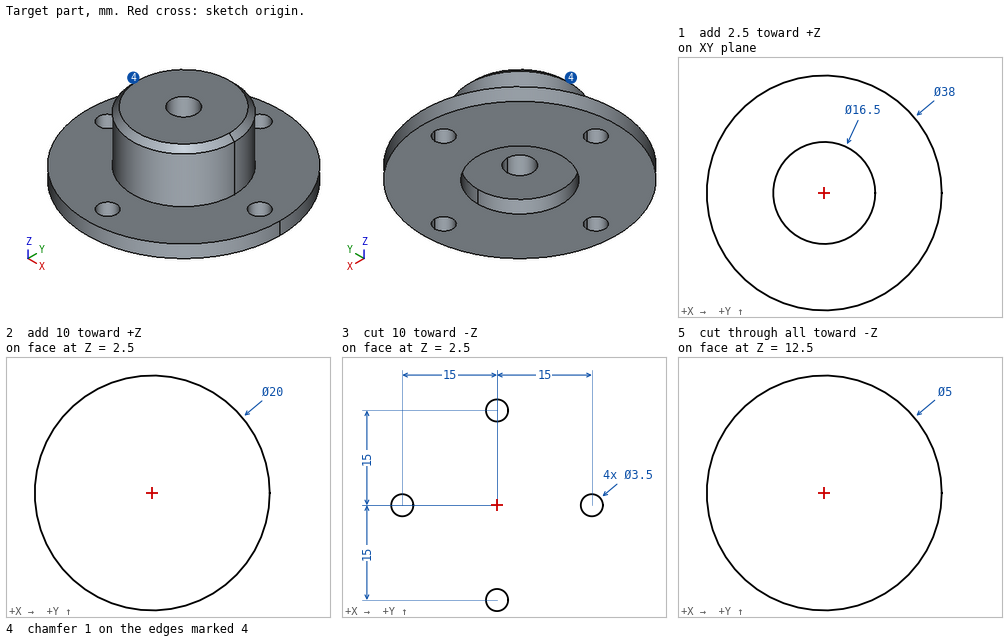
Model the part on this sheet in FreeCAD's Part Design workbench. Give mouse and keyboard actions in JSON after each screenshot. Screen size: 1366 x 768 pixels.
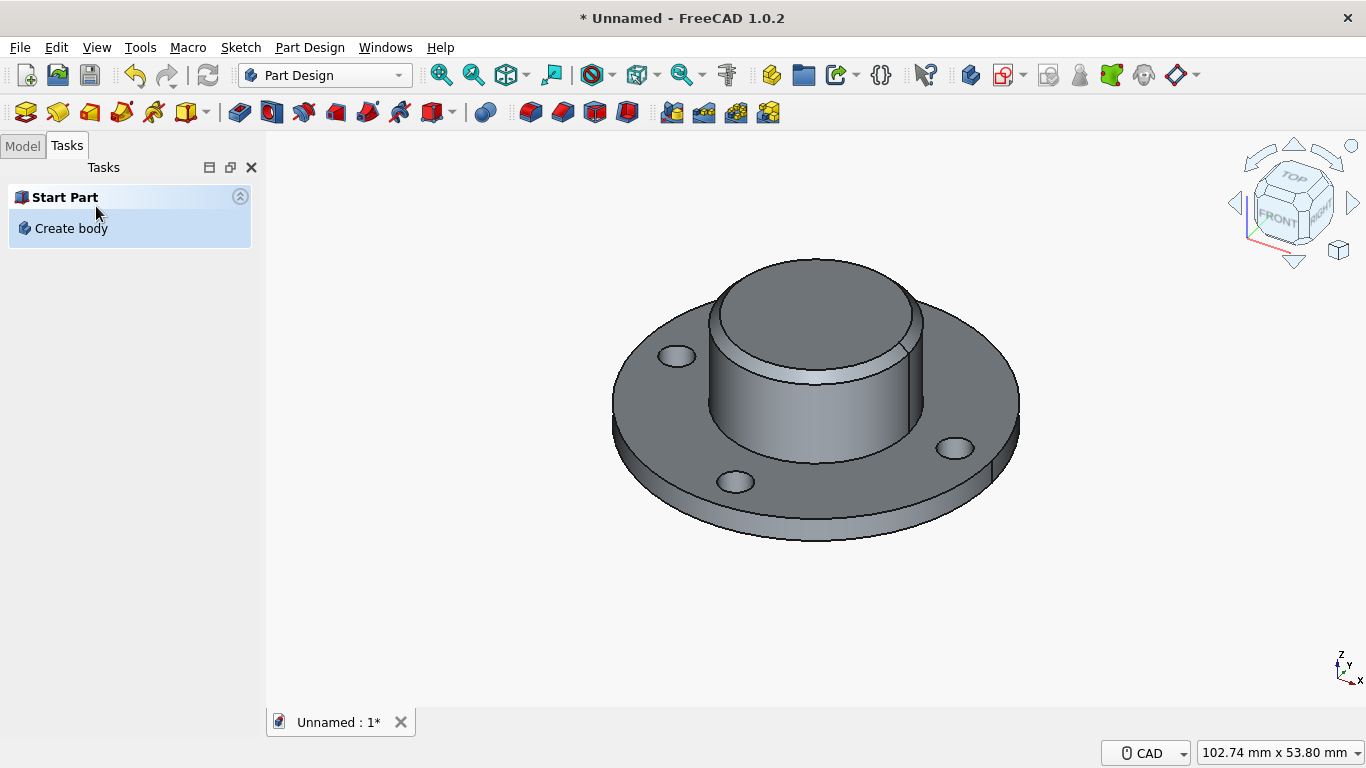
{"action": "left_click", "coordinate": [816, 314]}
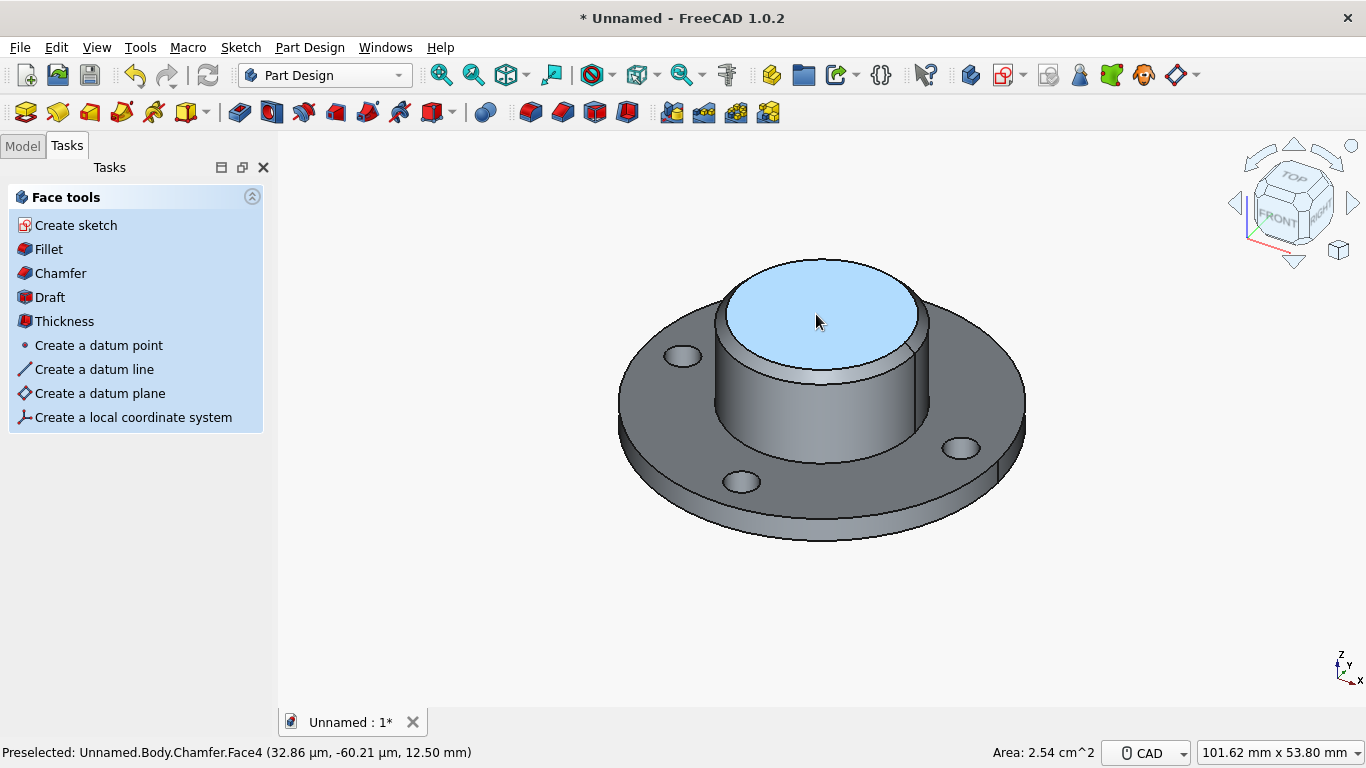
{"action": "left_click", "coordinate": [1004, 76]}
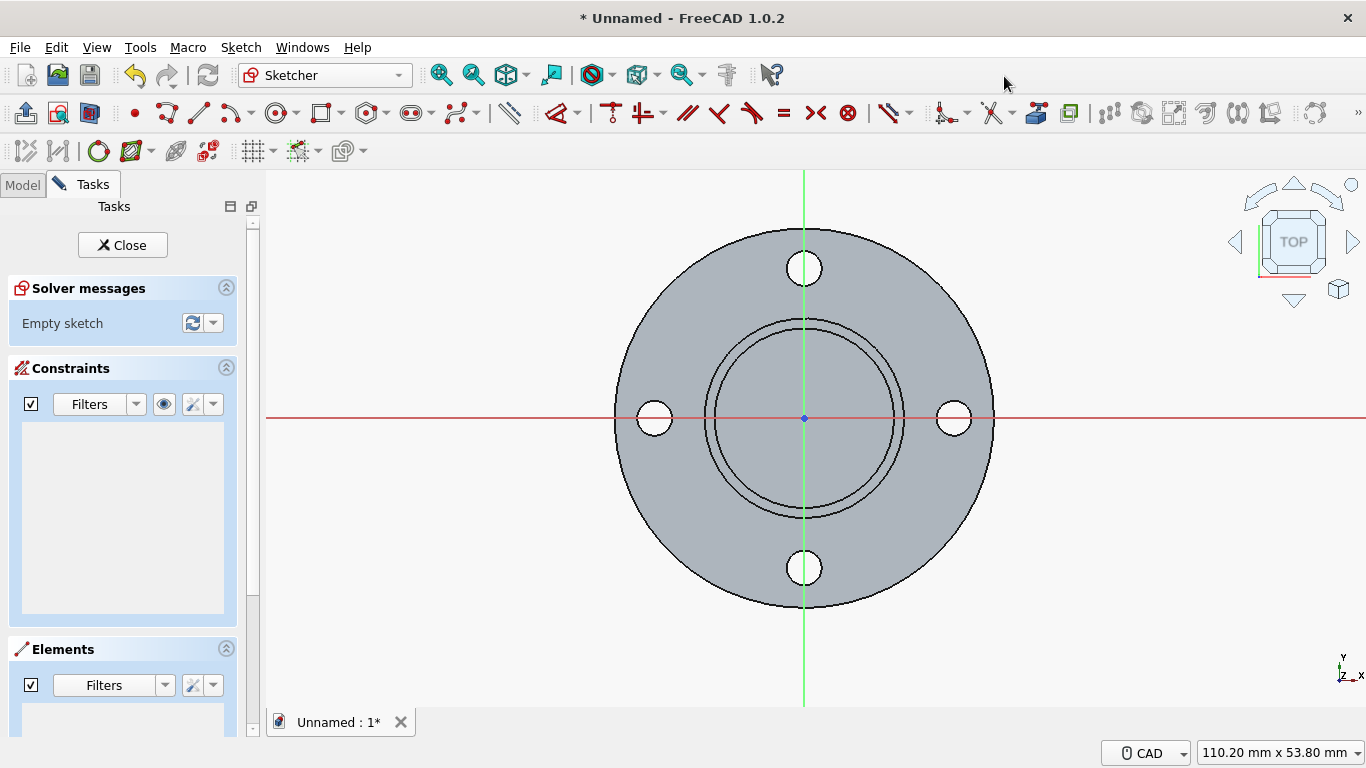
{"action": "scroll", "coordinate": [813, 415], "scroll_direction": "up", "scroll_amount": 10}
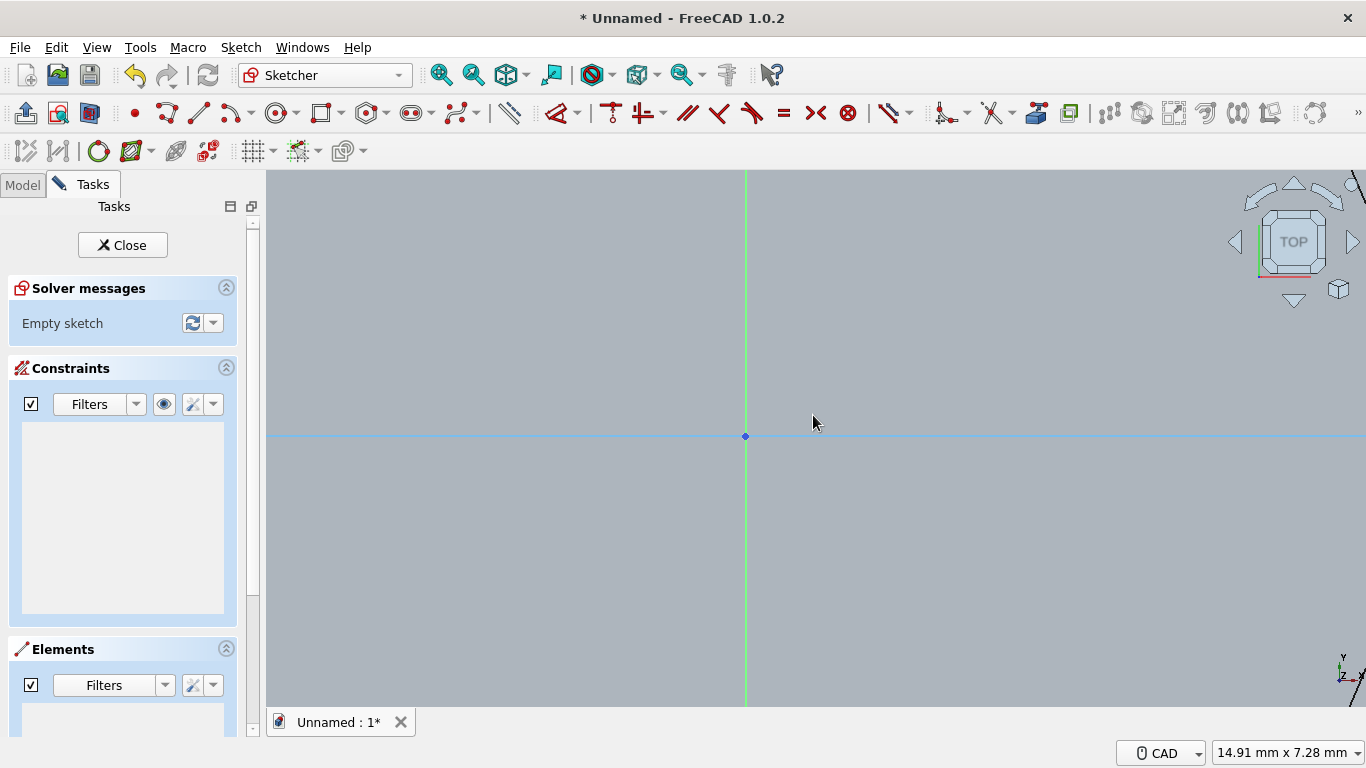
{"action": "key", "text": "g c"}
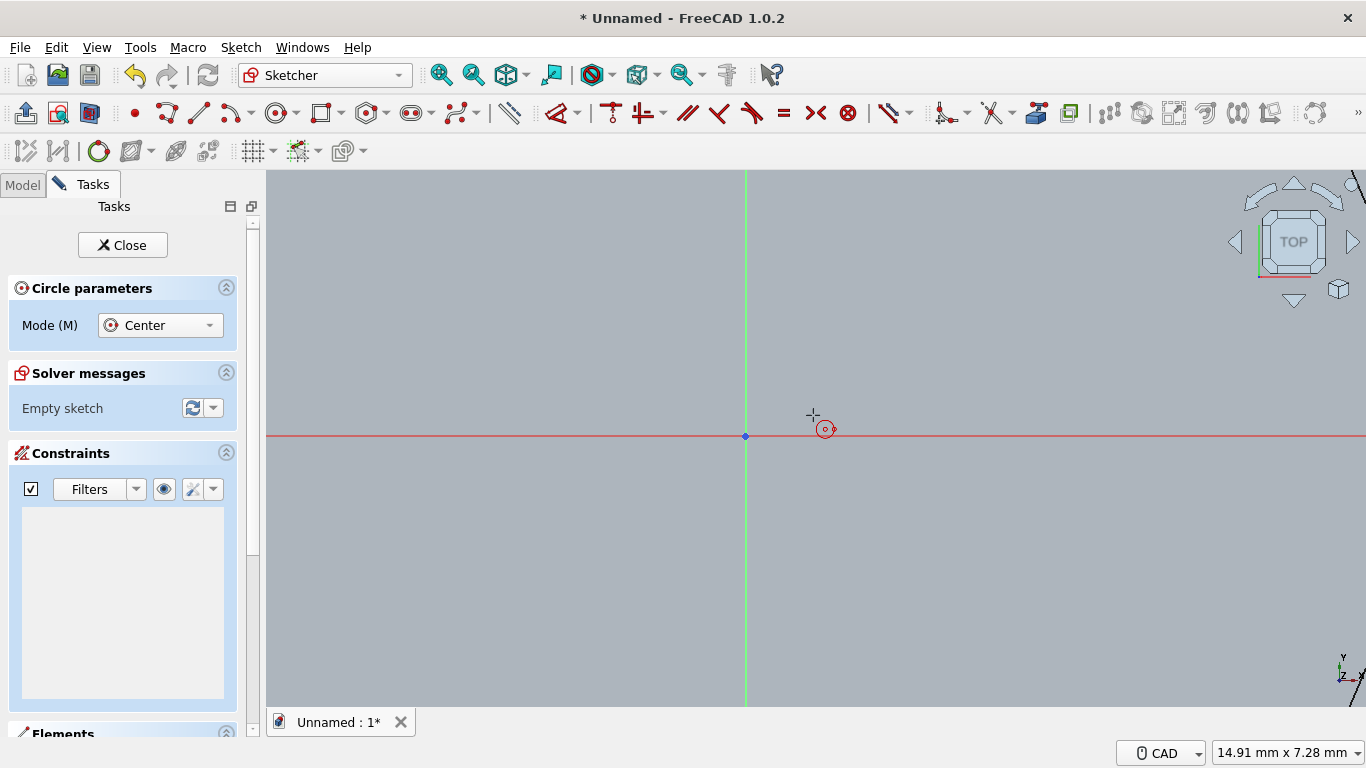
{"action": "left_click", "coordinate": [746, 436]}
{"action": "mouse_move", "coordinate": [876, 306]}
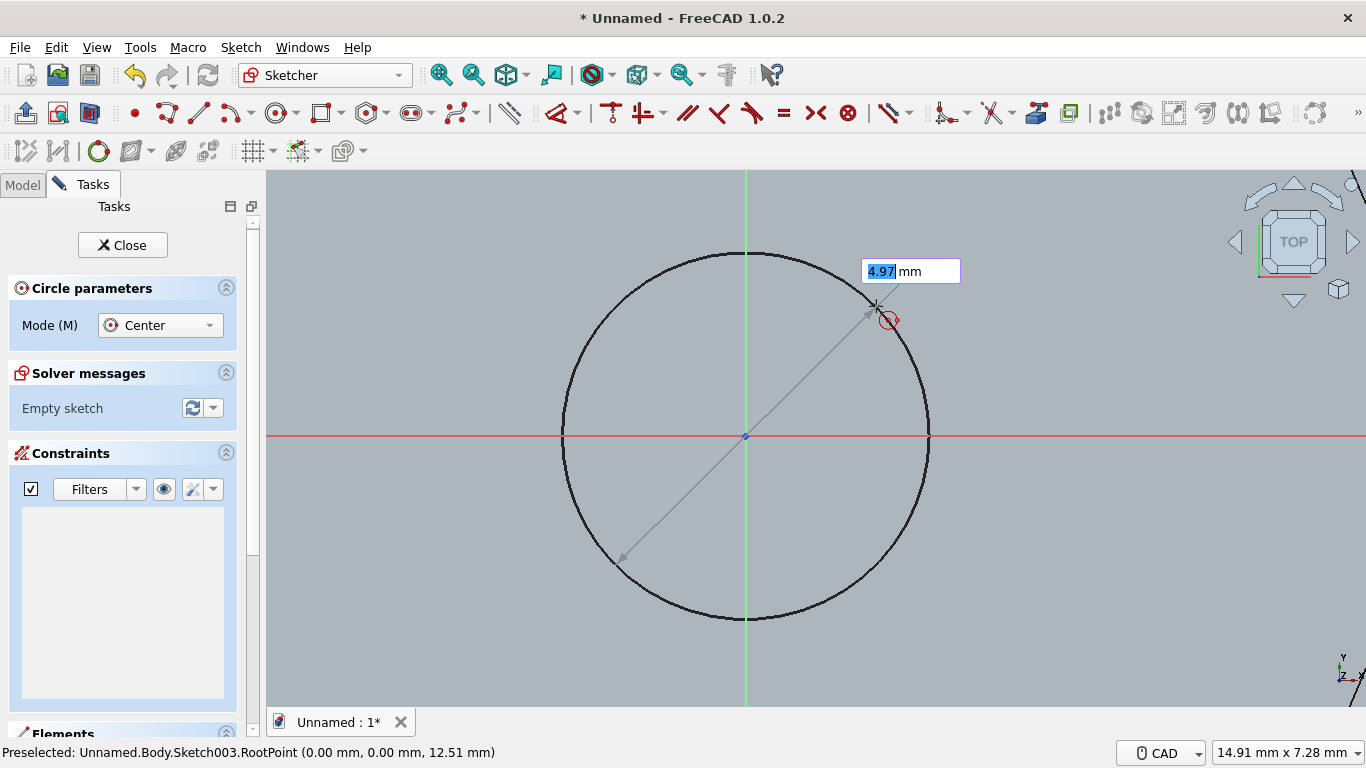
{"action": "type", "text": "5"}
{"action": "key", "text": "Return"}
{"action": "key", "text": "Escape"}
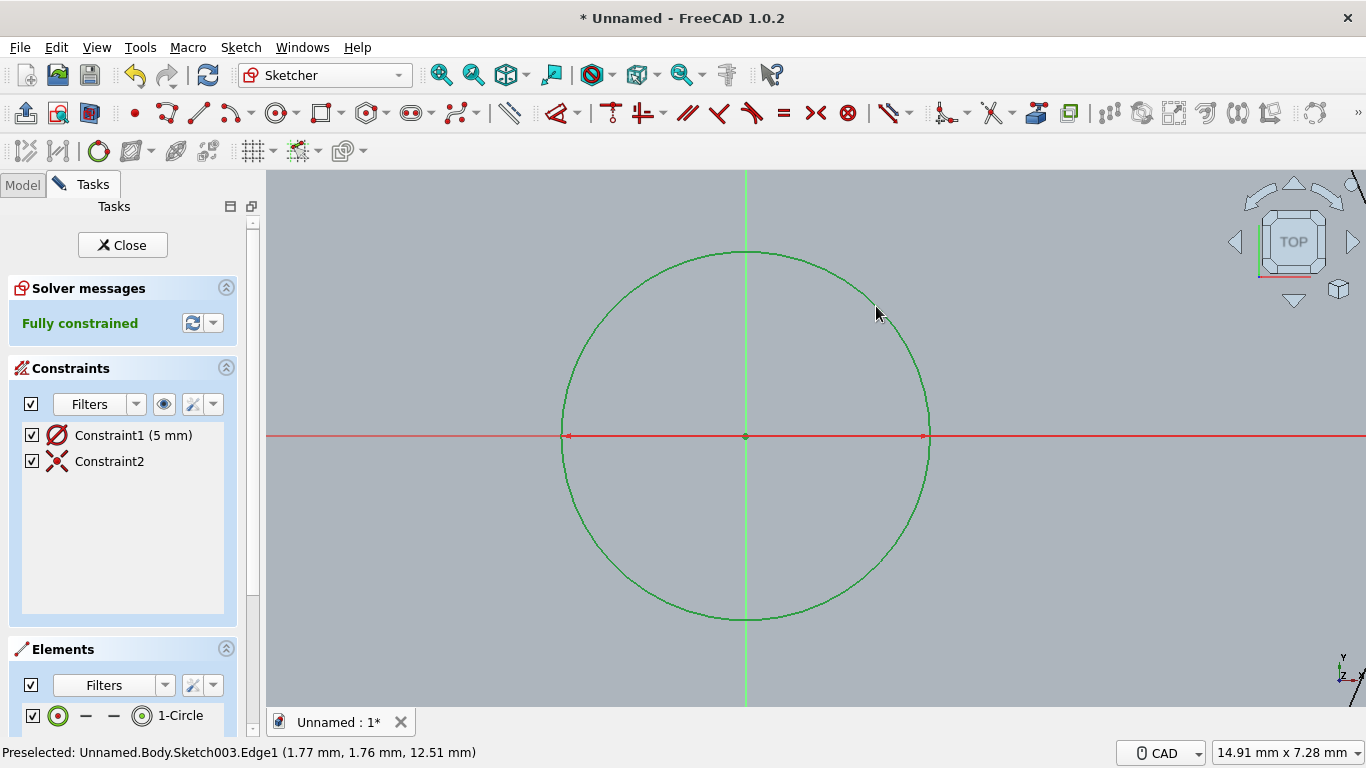
{"action": "left_click", "coordinate": [123, 245]}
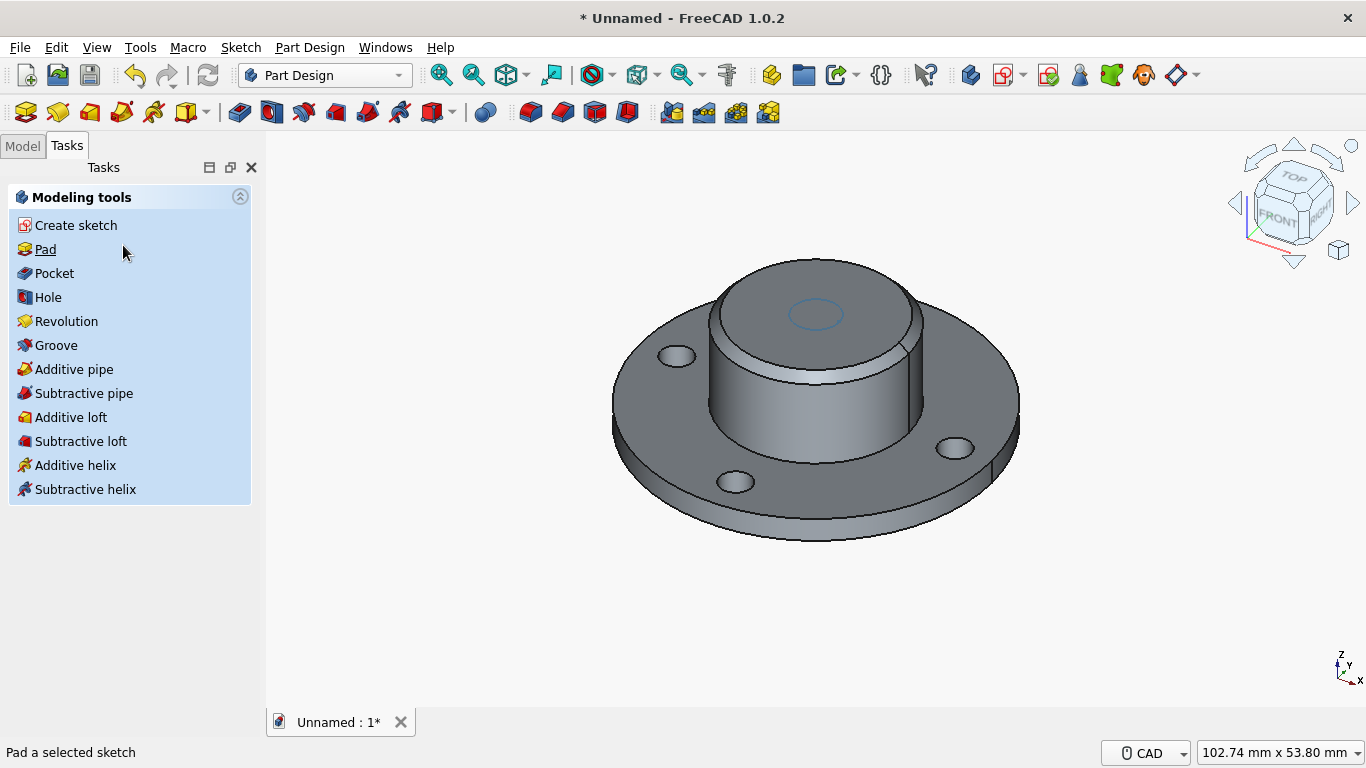
{"action": "left_click", "coordinate": [240, 112]}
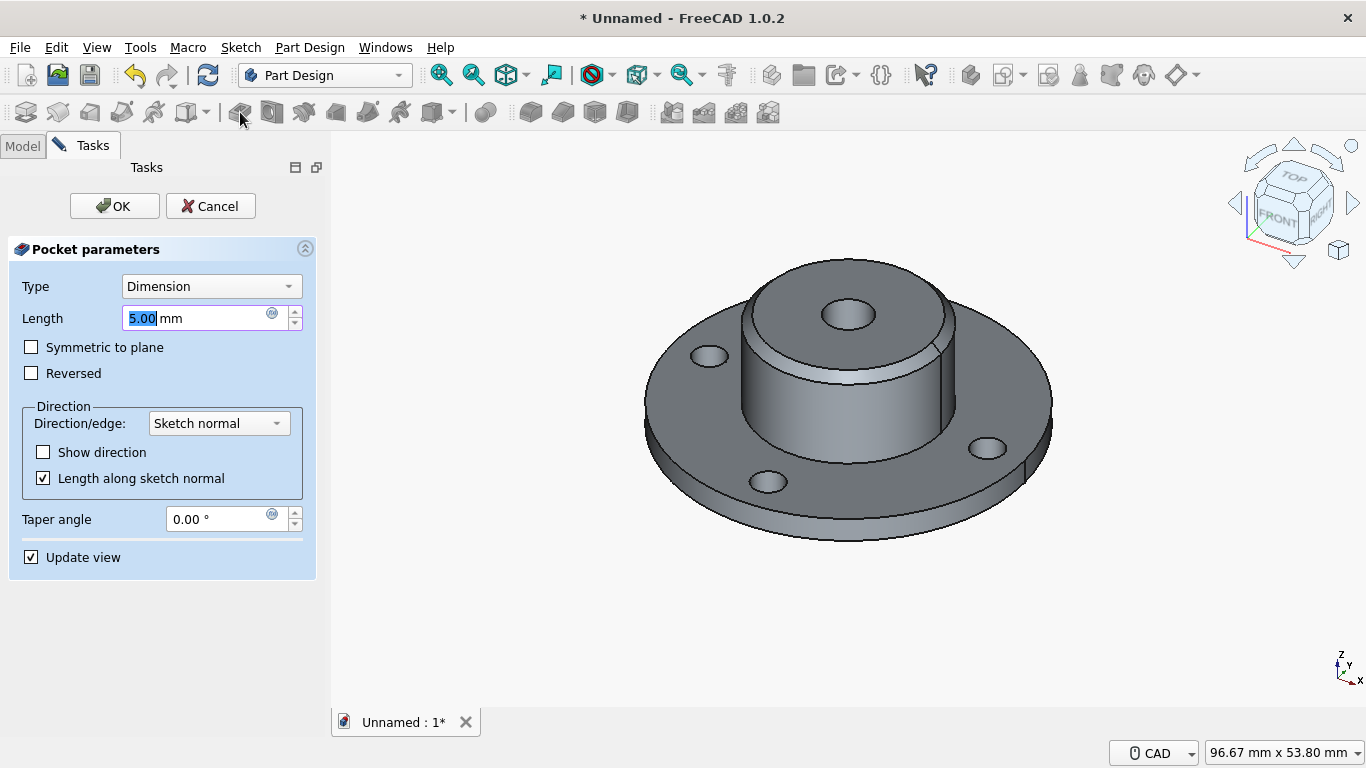
{"action": "left_click", "coordinate": [212, 286]}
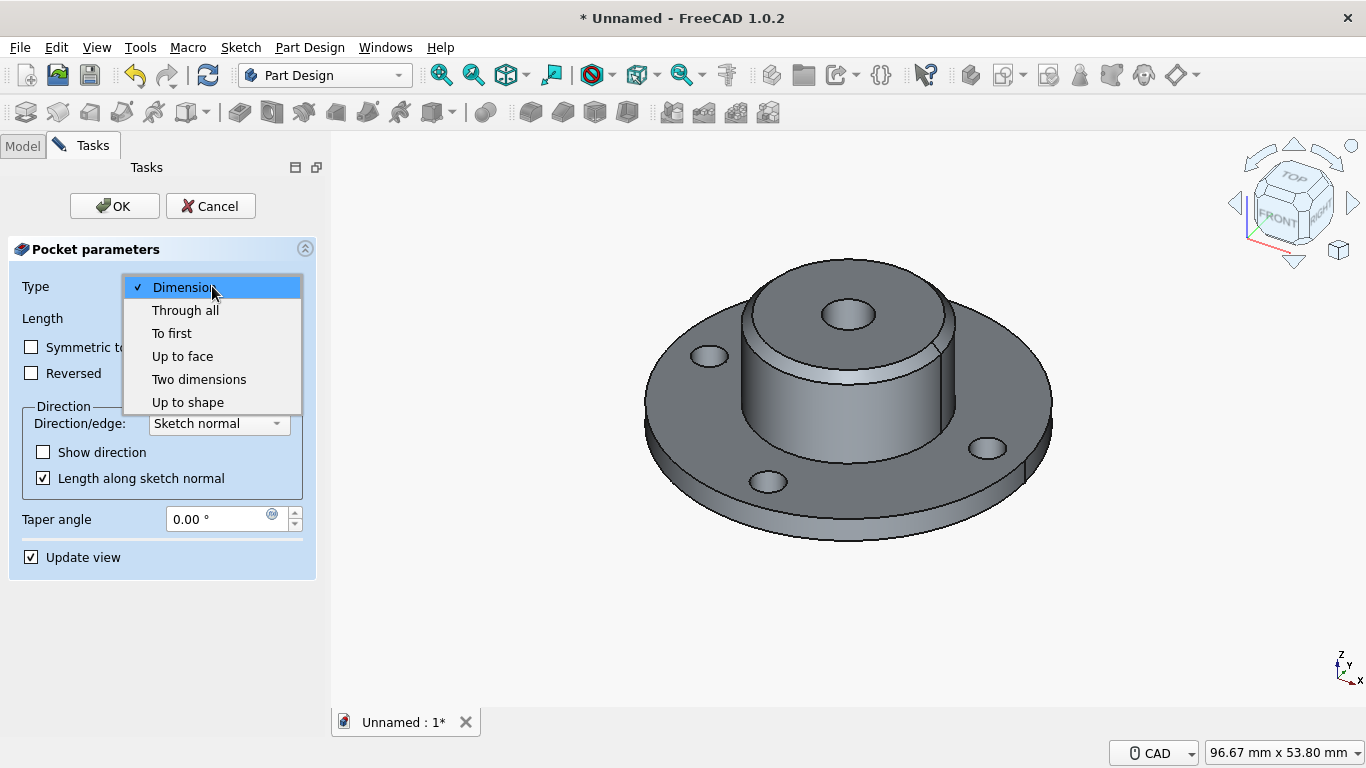
{"action": "left_click", "coordinate": [212, 310]}